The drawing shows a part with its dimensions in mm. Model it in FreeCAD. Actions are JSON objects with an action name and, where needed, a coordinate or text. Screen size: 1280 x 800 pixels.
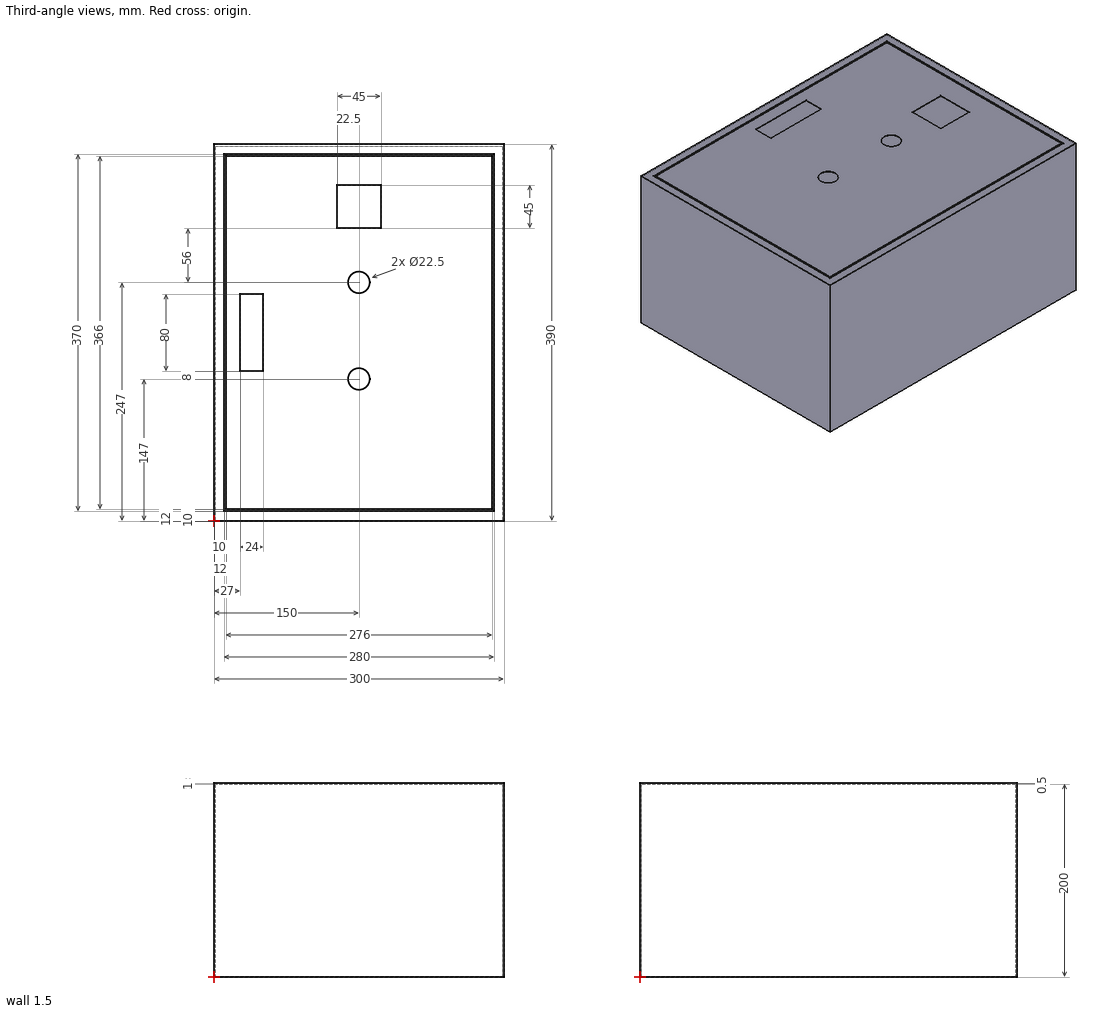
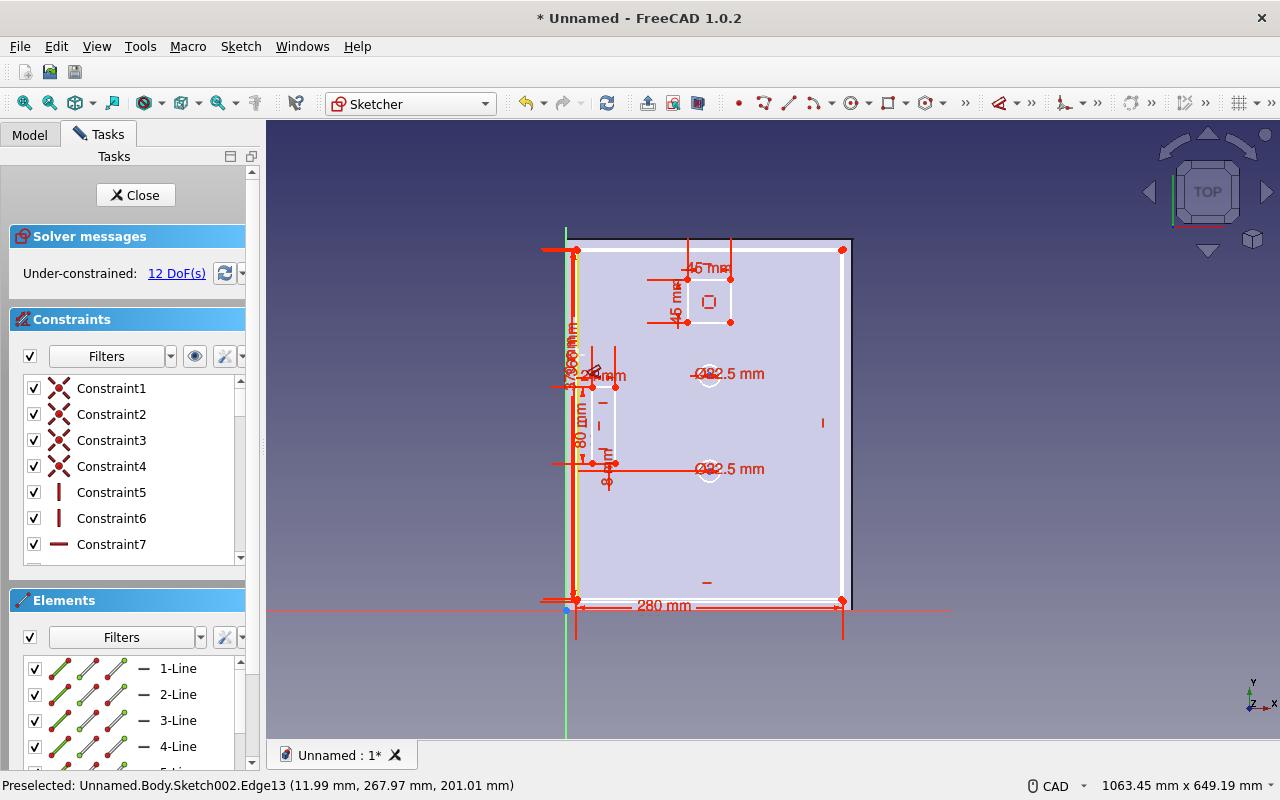
{"action": "scroll", "coordinate": [657, 599], "scroll_direction": "up", "scroll_amount": 9}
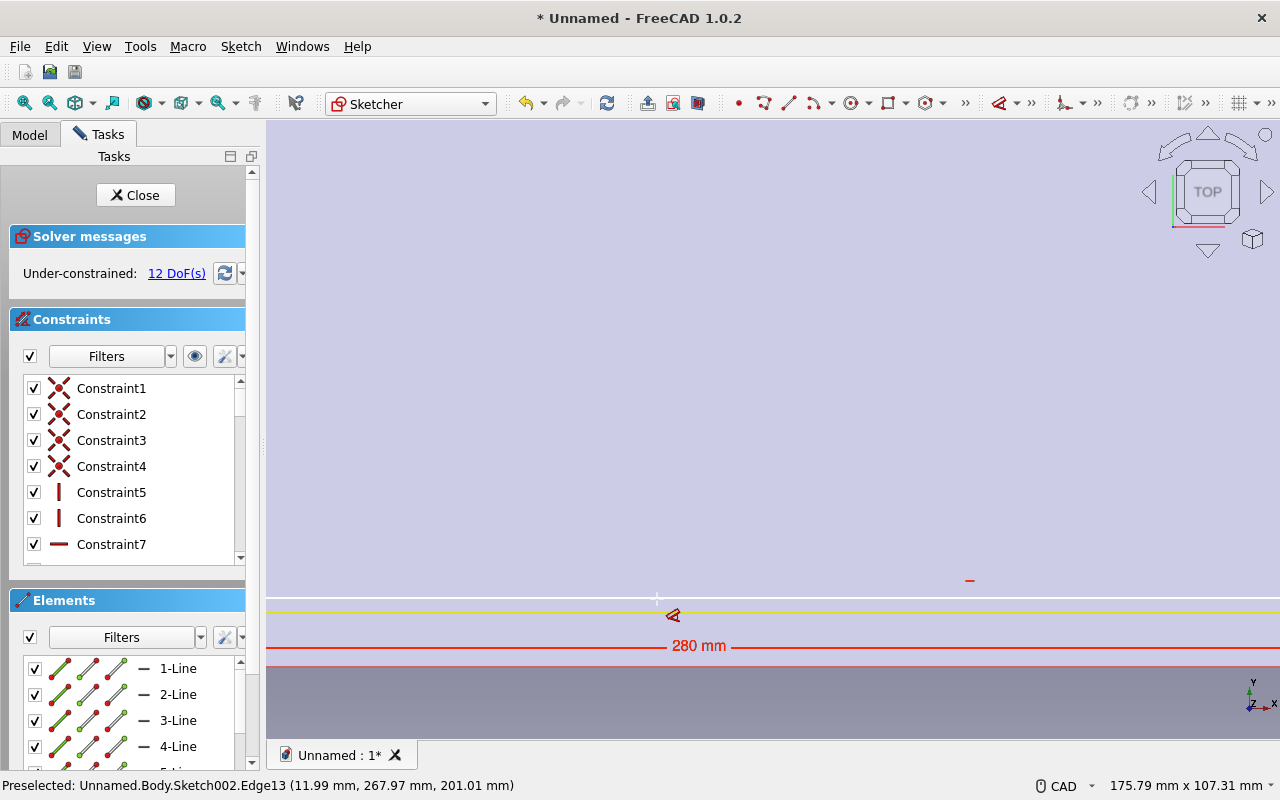
{"action": "left_click", "coordinate": [654, 598]}
{"action": "left_click", "coordinate": [516, 632]}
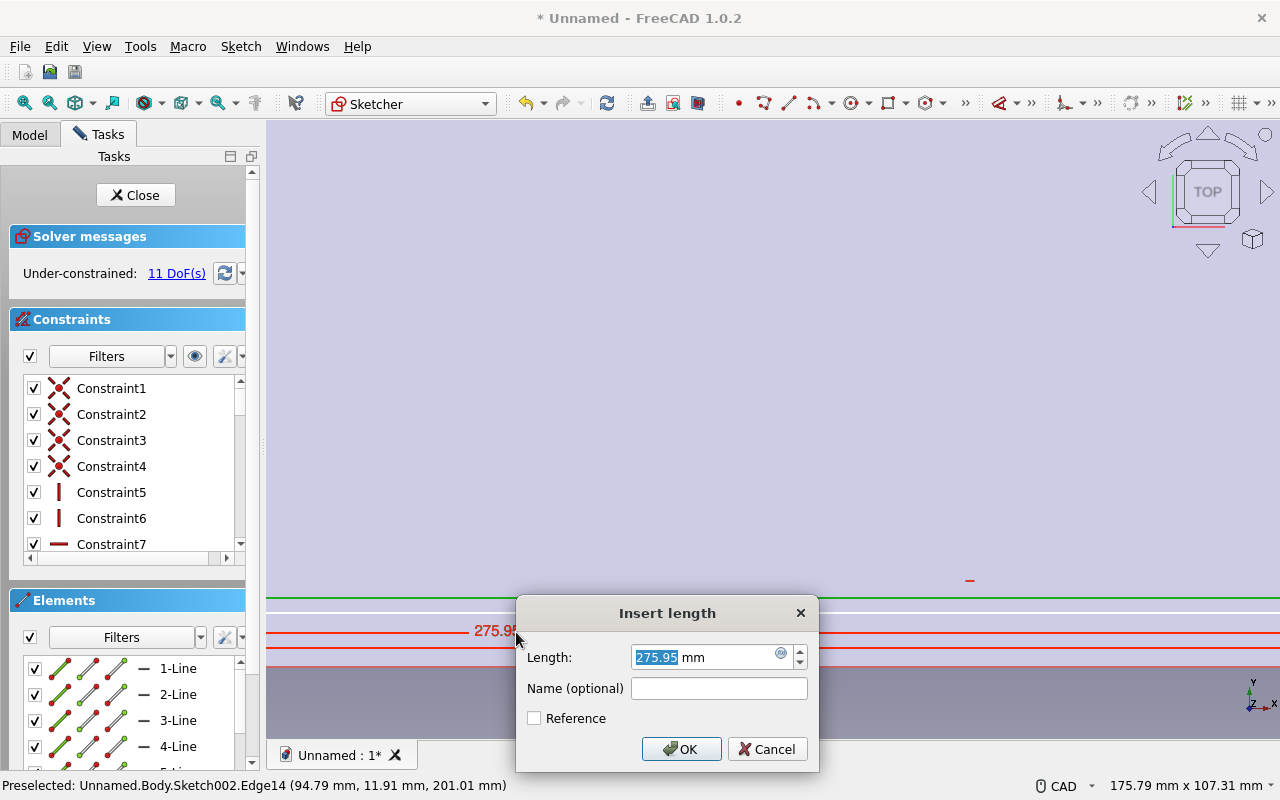
{"action": "type", "text": "276"}
{"action": "key", "text": "Return"}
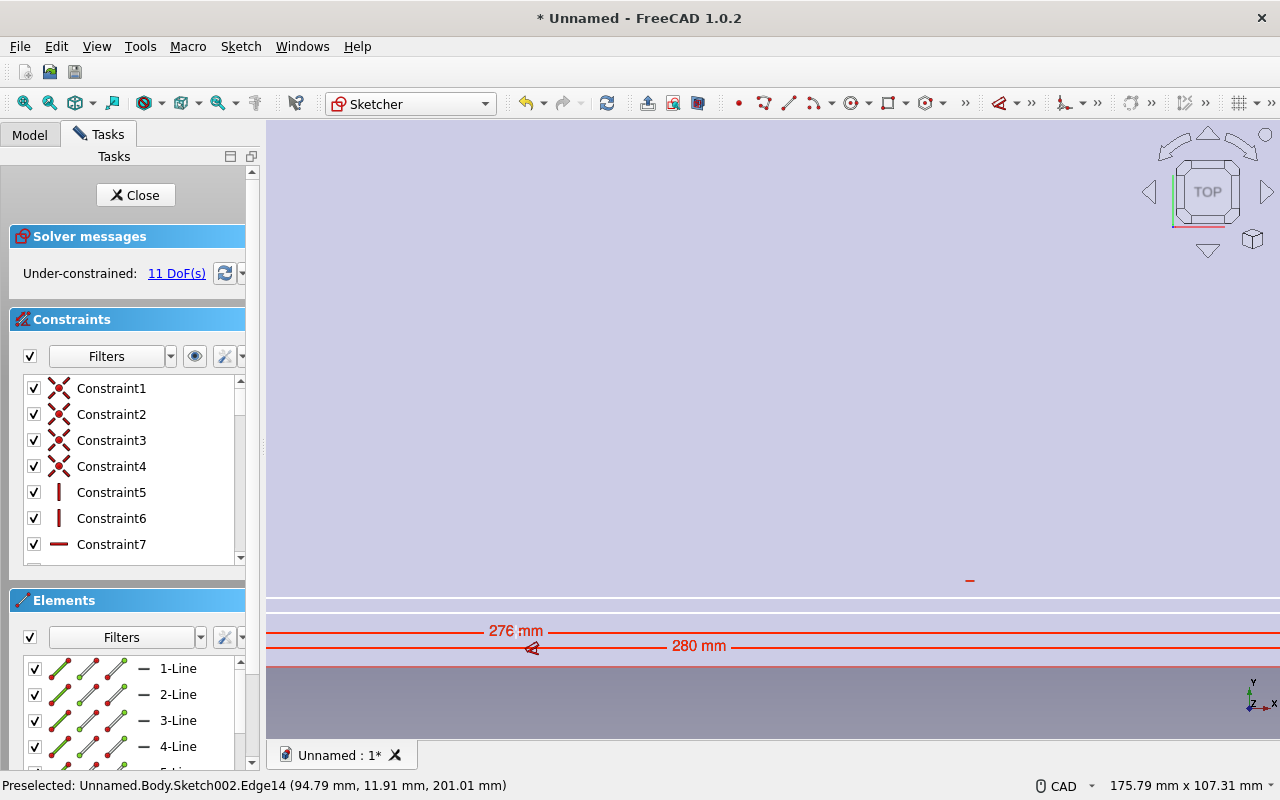
{"action": "scroll", "coordinate": [657, 600], "scroll_direction": "down", "scroll_amount": 9}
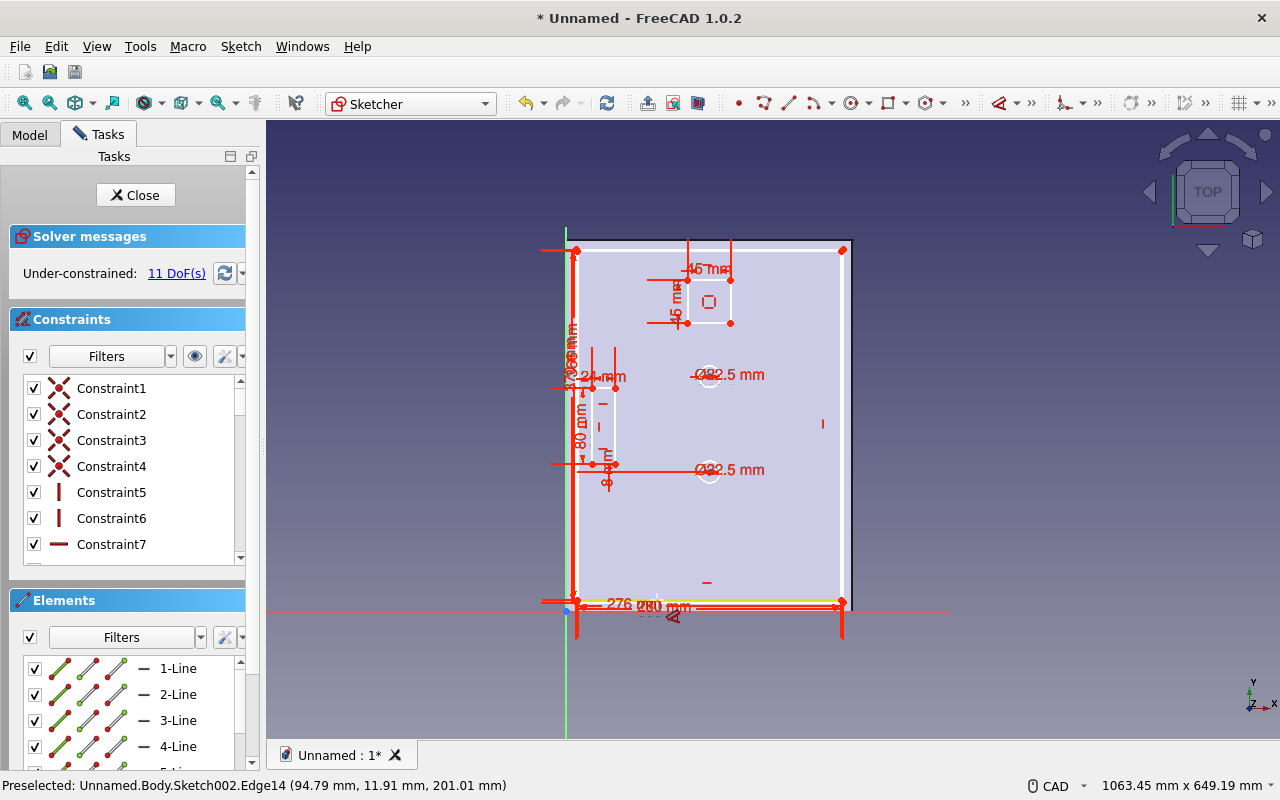
{"action": "scroll", "coordinate": [576, 250], "scroll_direction": "up", "scroll_amount": 9}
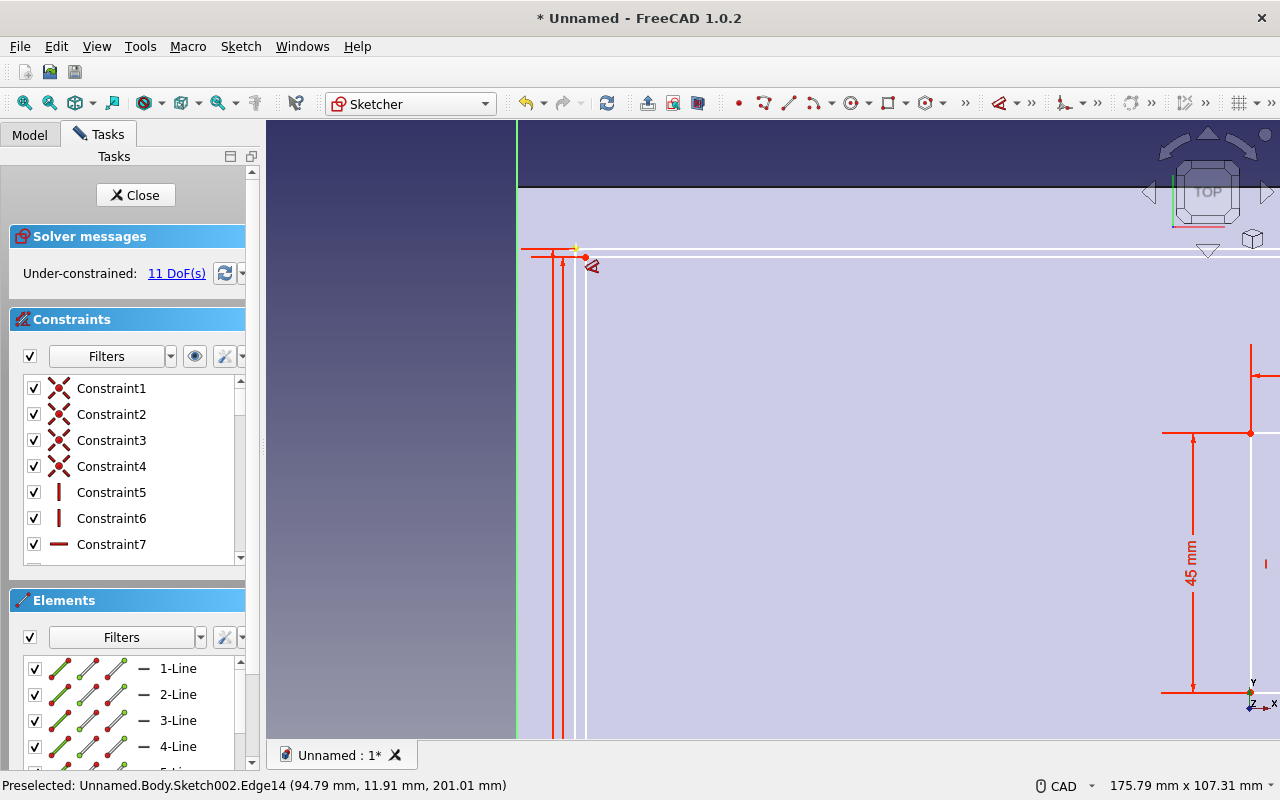
{"action": "left_click", "coordinate": [575, 249]}
{"action": "left_click", "coordinate": [546, 215]}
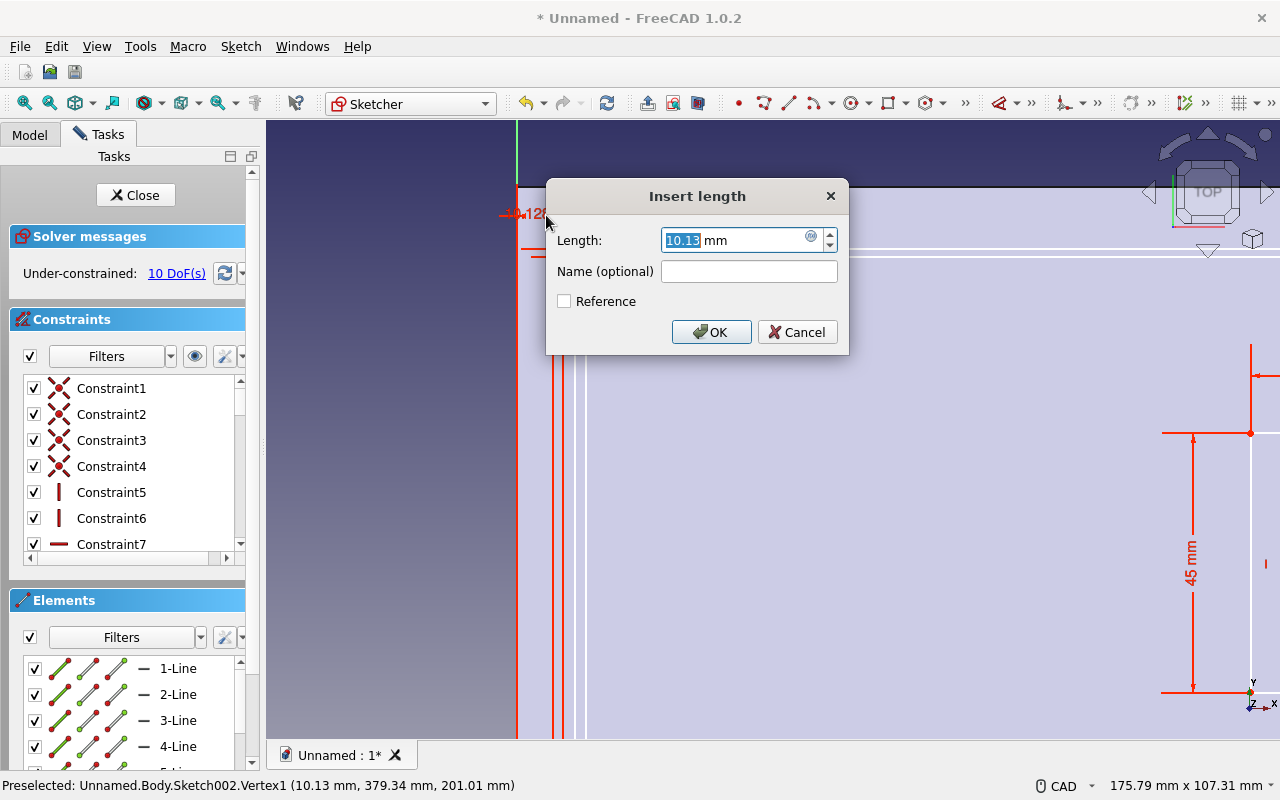
{"action": "type", "text": "10"}
{"action": "key", "text": "Return"}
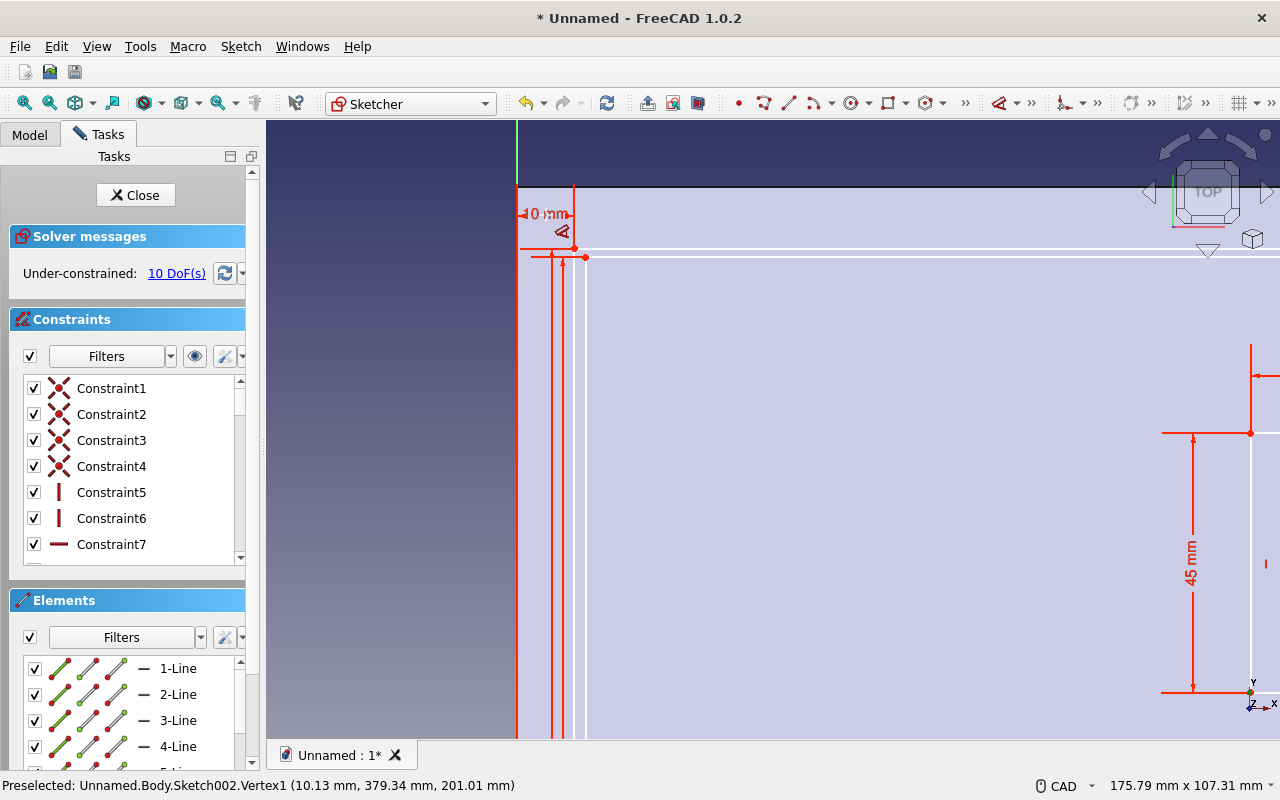
{"action": "scroll", "coordinate": [576, 249], "scroll_direction": "down", "scroll_amount": 9}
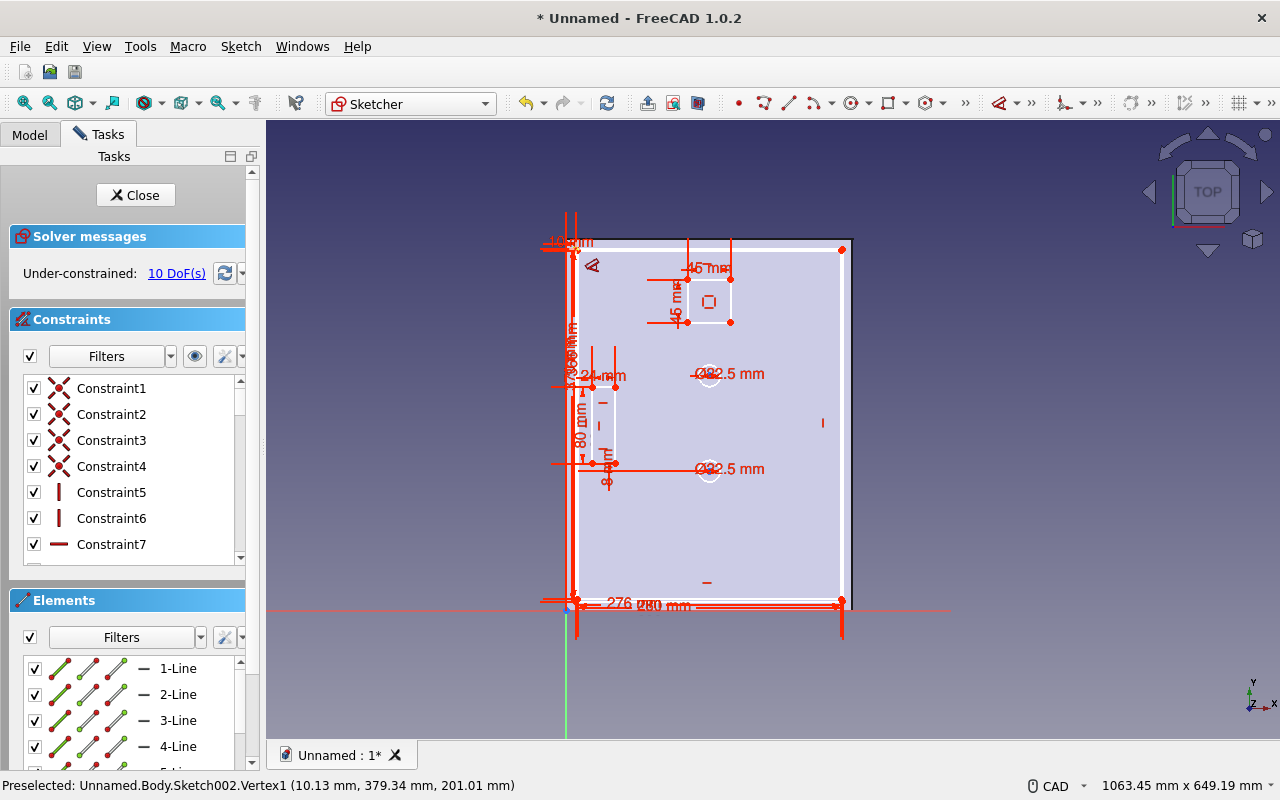
{"action": "scroll", "coordinate": [576, 602], "scroll_direction": "up", "scroll_amount": 8}